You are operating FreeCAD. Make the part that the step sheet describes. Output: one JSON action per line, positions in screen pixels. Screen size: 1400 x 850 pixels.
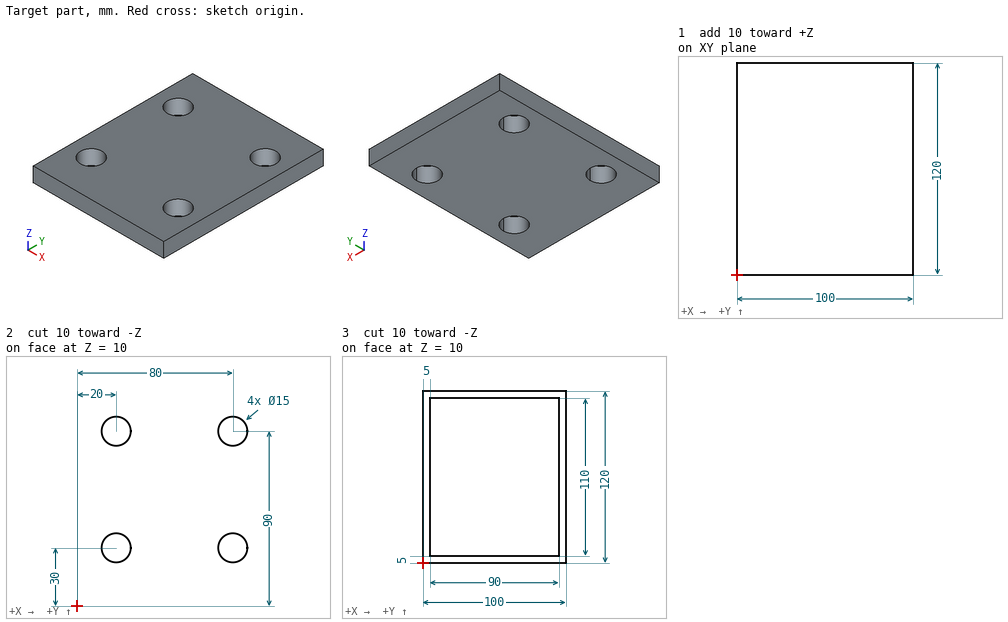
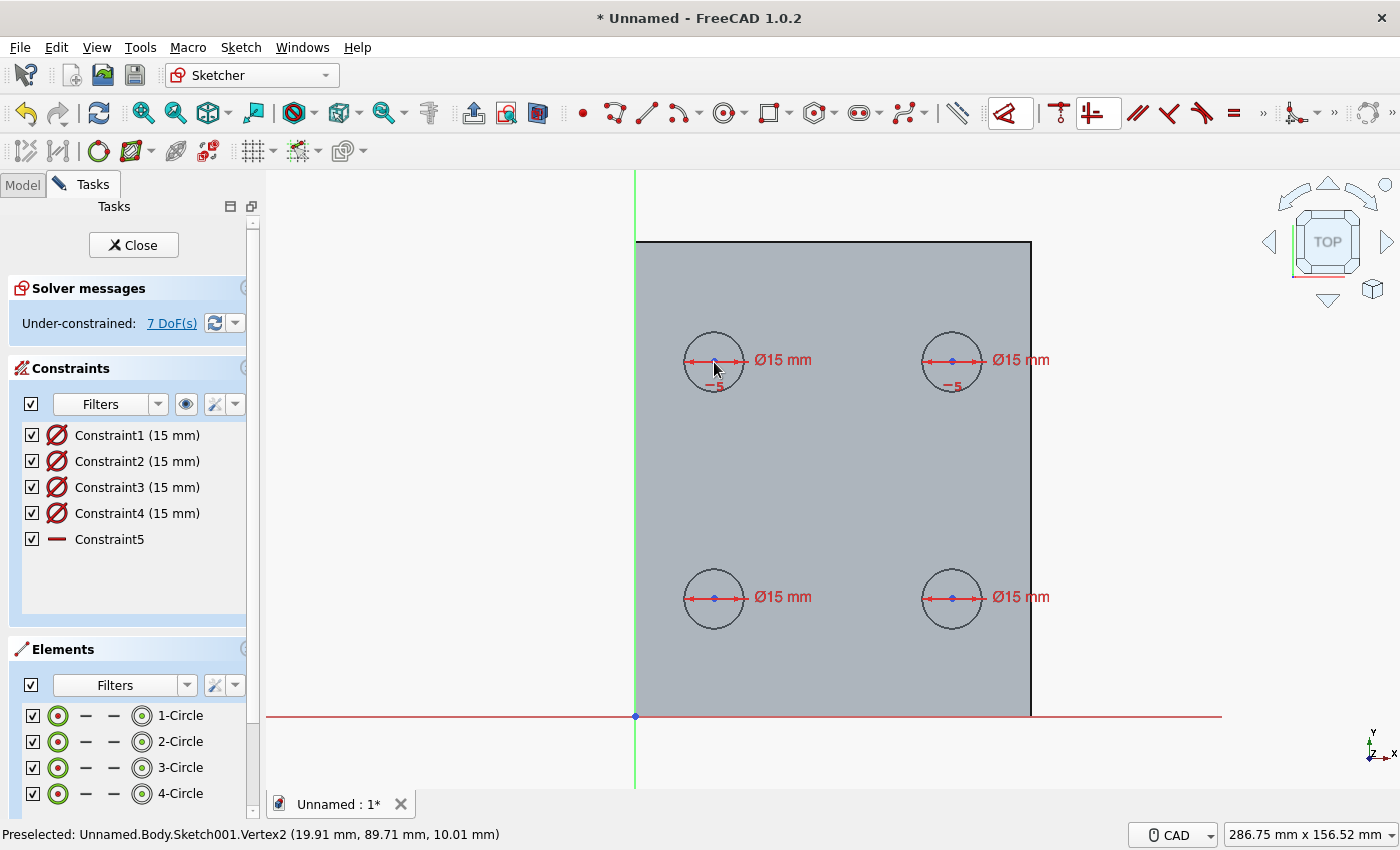
{"action": "left_click", "coordinate": [714, 362]}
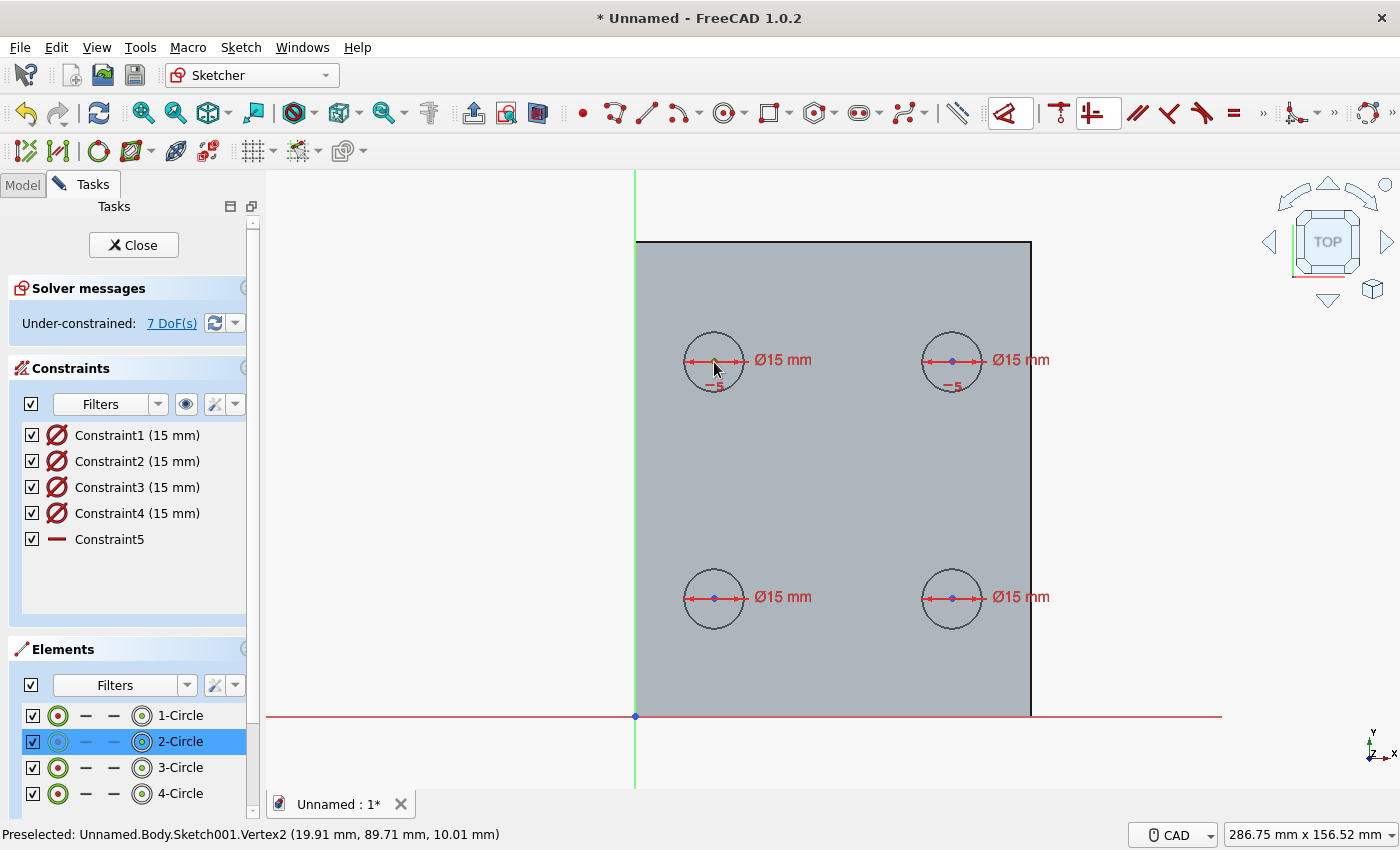
{"action": "left_click", "coordinate": [714, 599]}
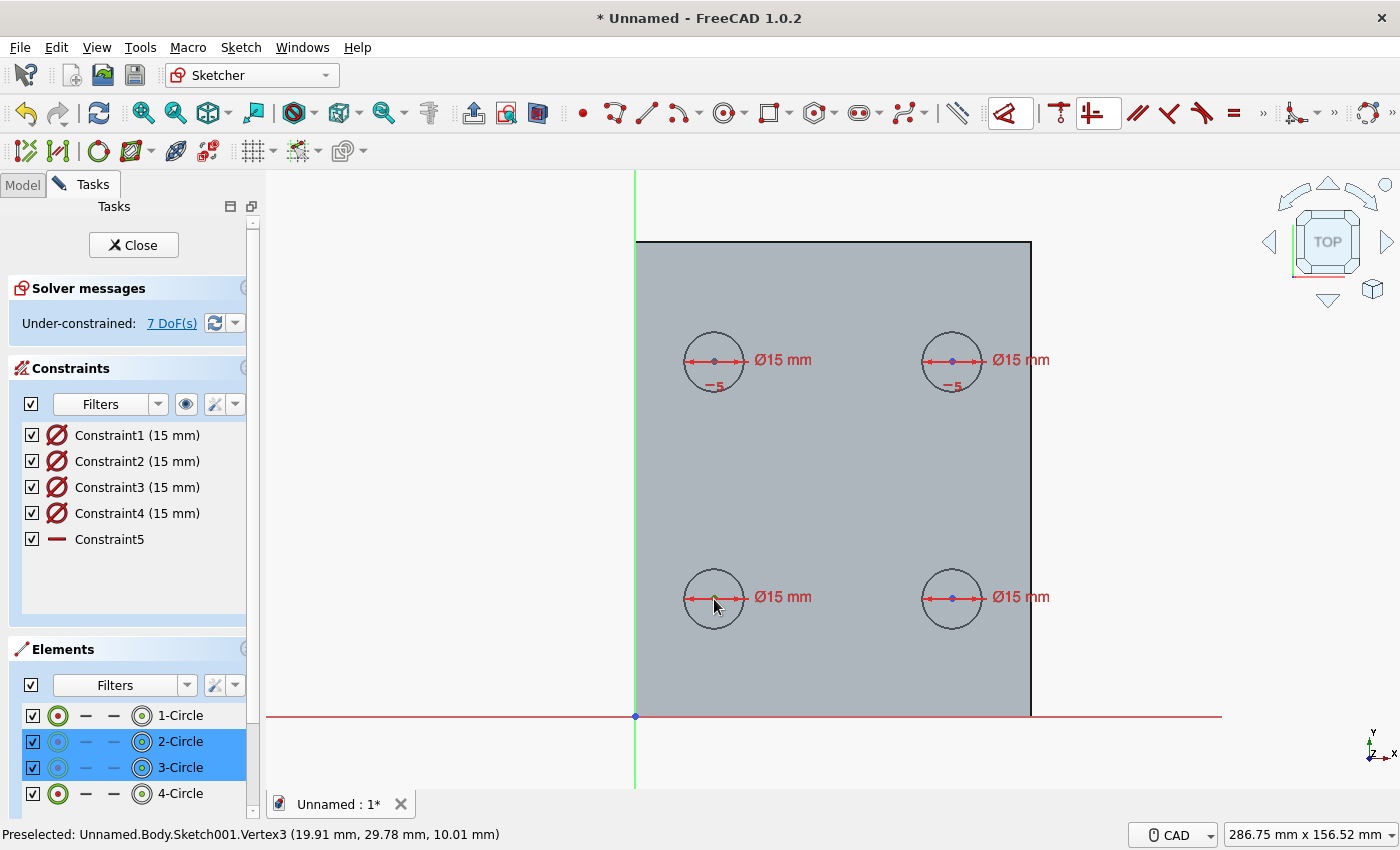
{"action": "key", "text": "v"}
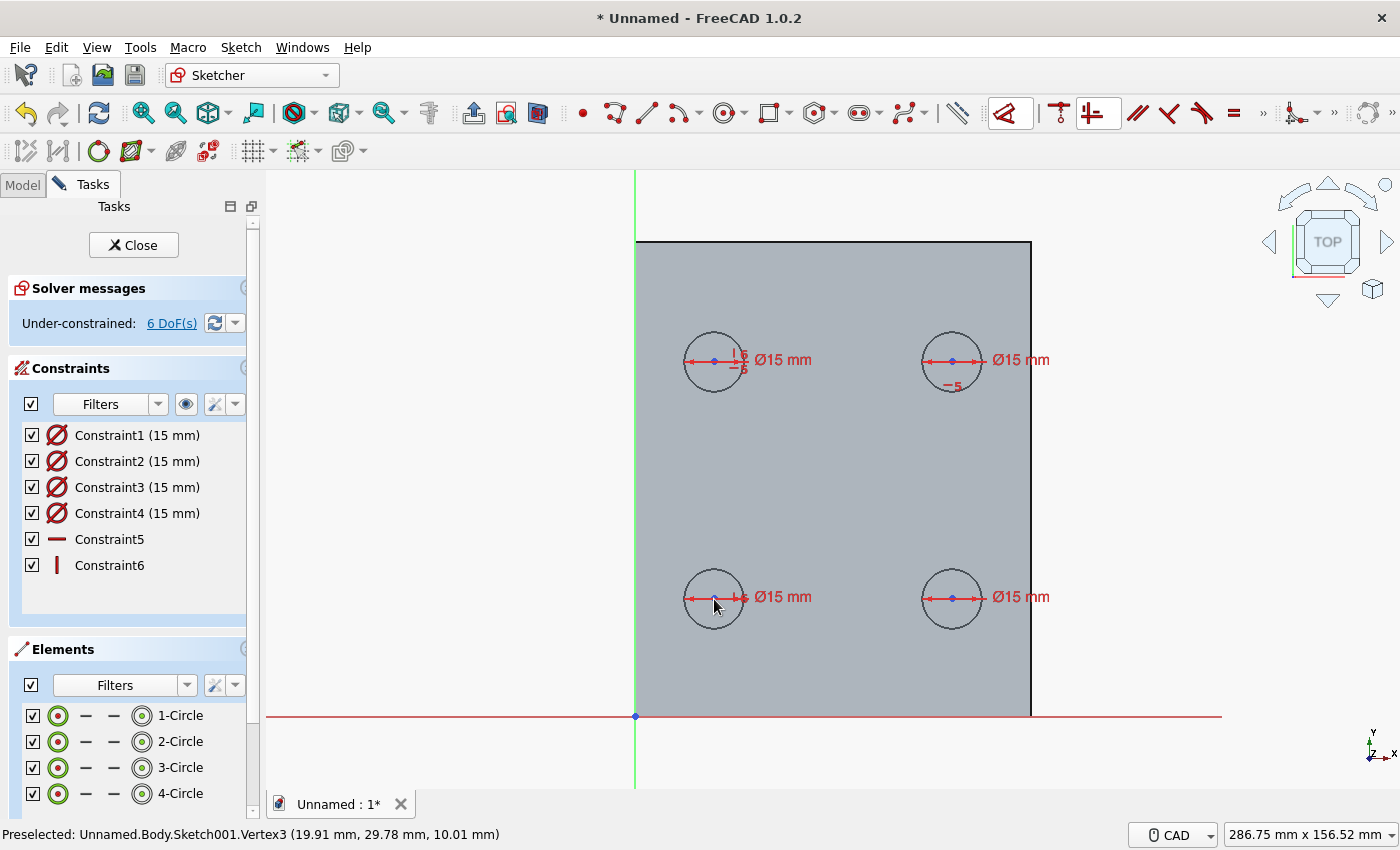
{"action": "left_click", "coordinate": [952, 362]}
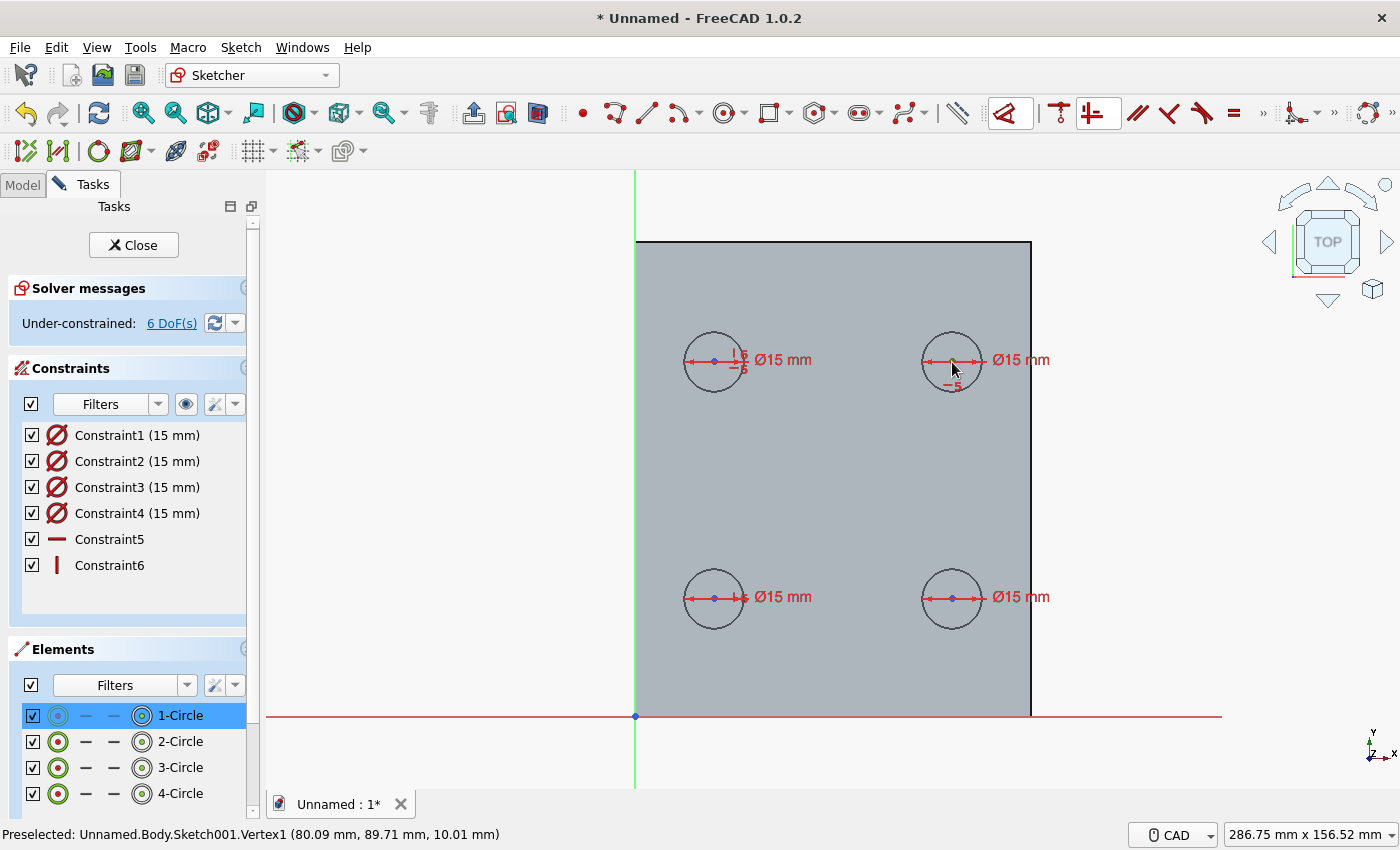
{"action": "left_click", "coordinate": [952, 599]}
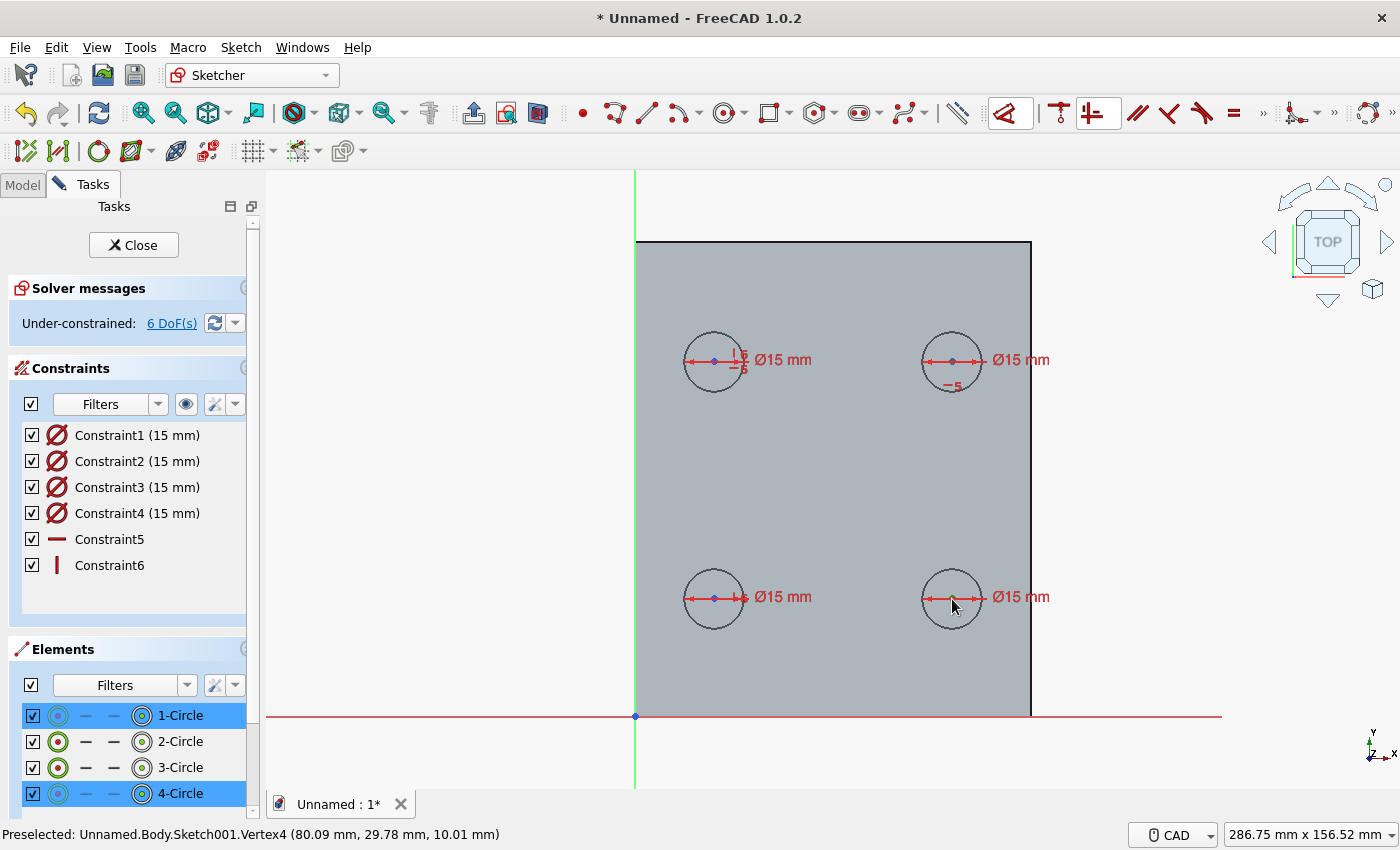
{"action": "key", "text": "v"}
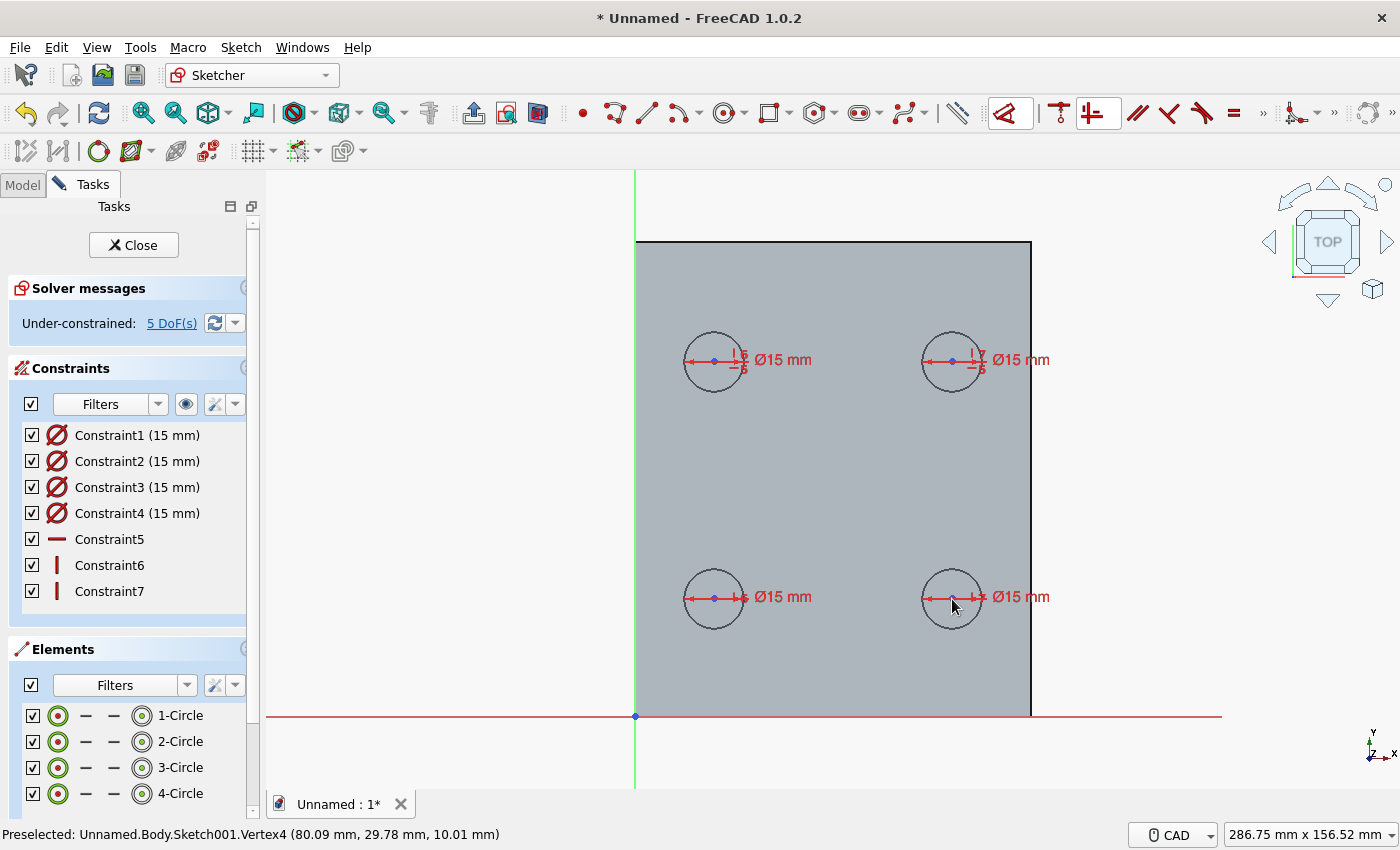
{"action": "left_click", "coordinate": [714, 599]}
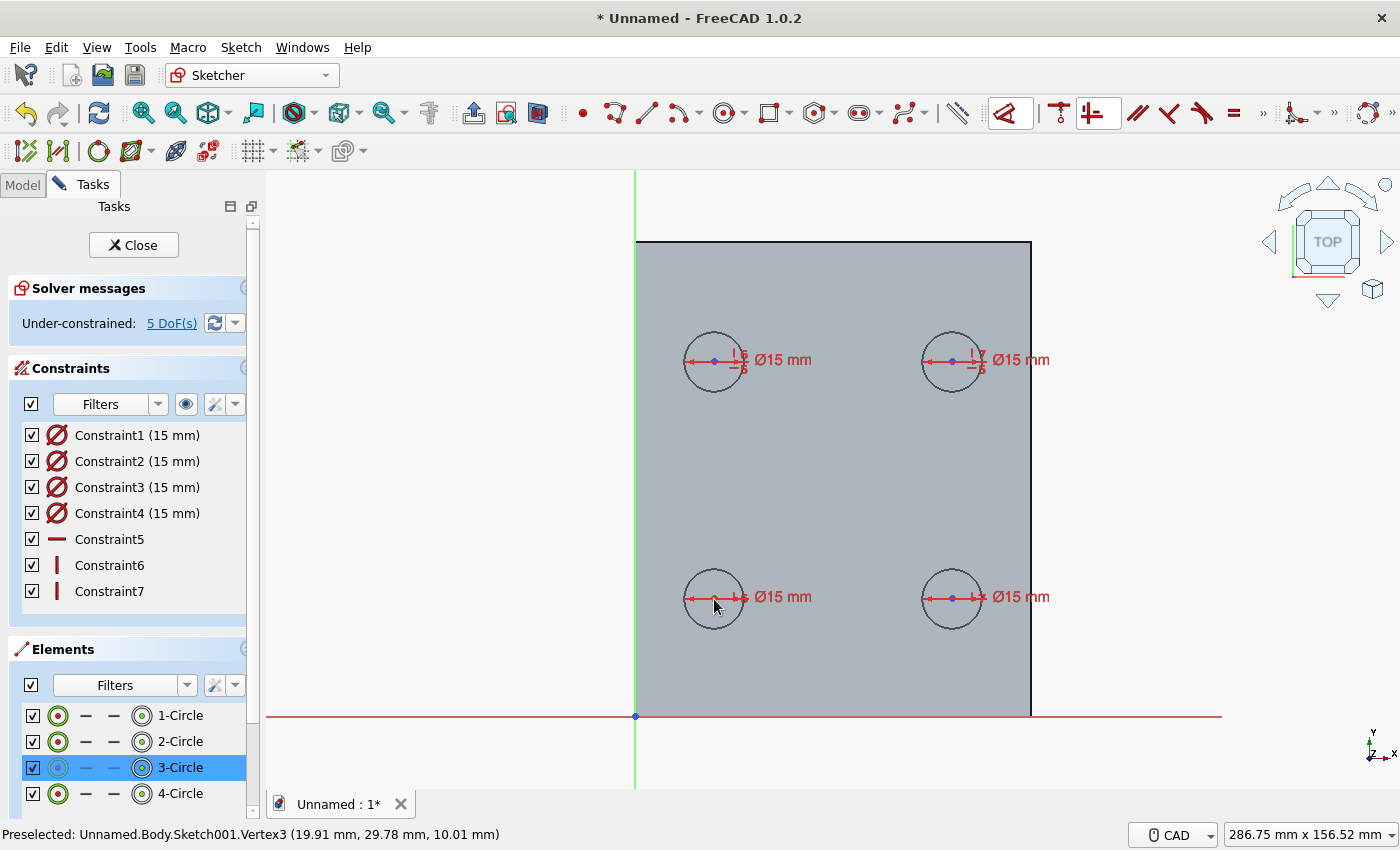
{"action": "left_click", "coordinate": [952, 599]}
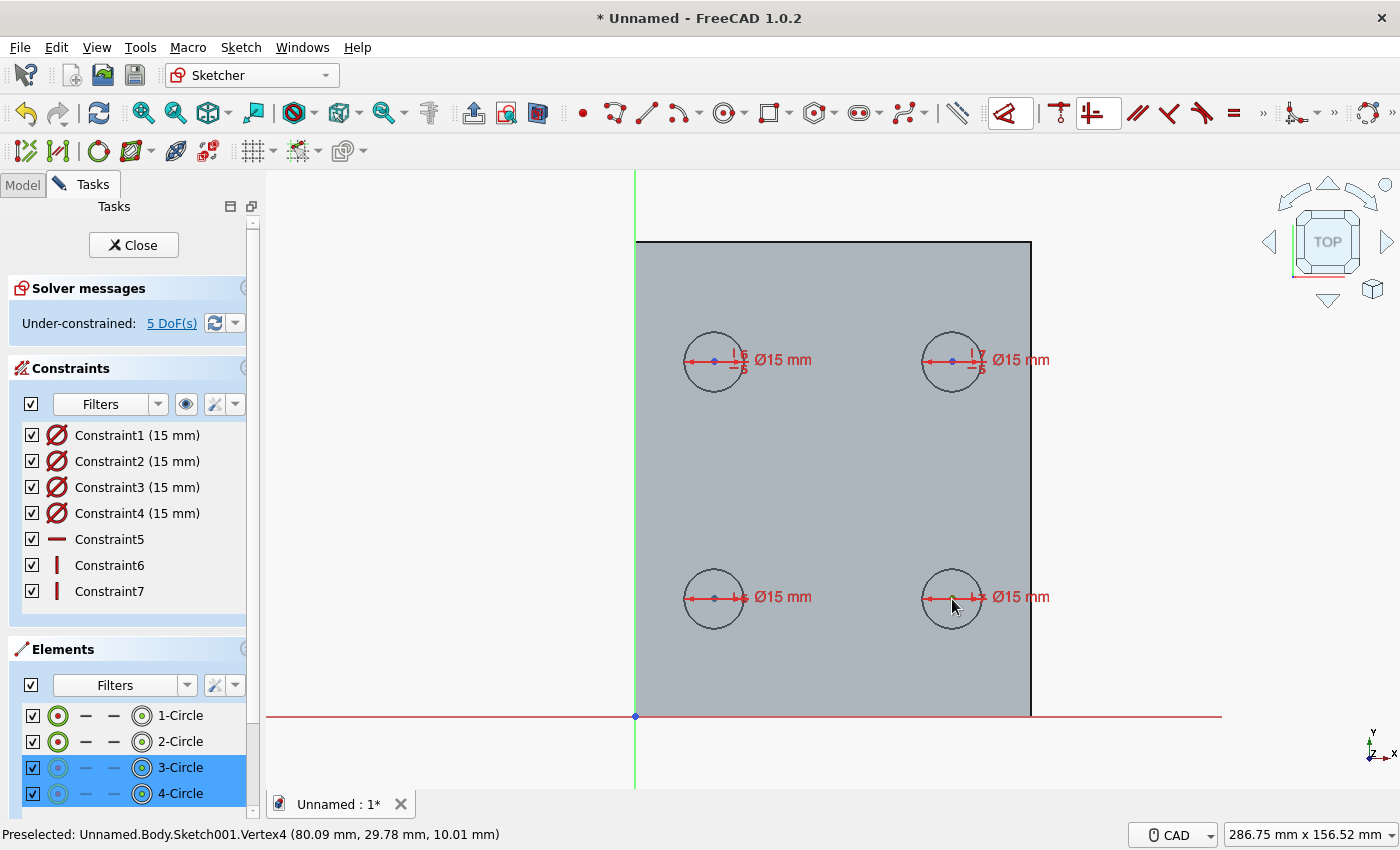
{"action": "key", "text": "h"}